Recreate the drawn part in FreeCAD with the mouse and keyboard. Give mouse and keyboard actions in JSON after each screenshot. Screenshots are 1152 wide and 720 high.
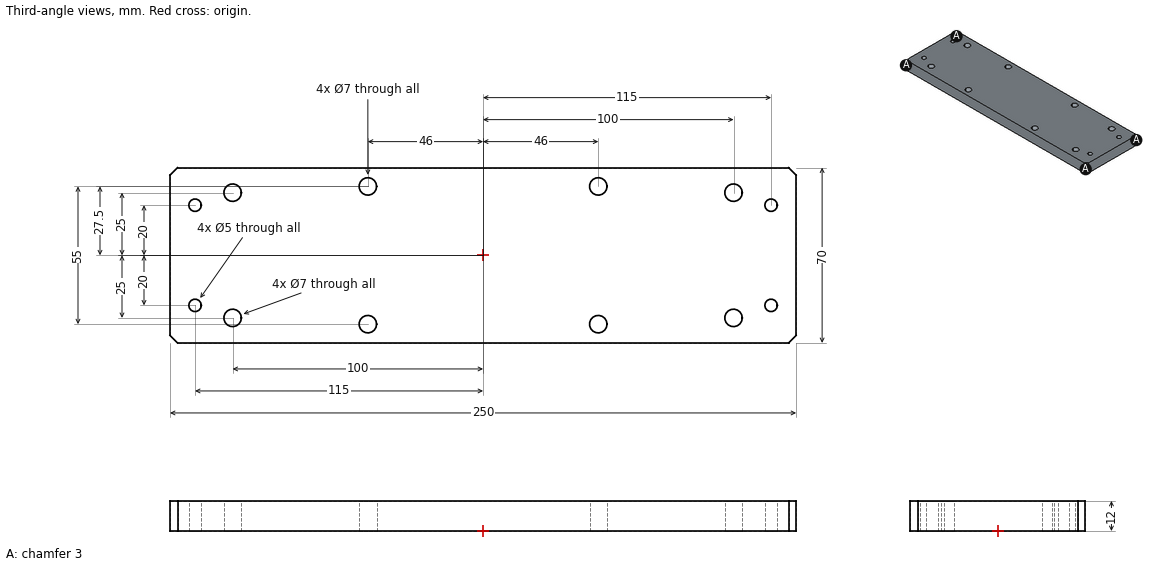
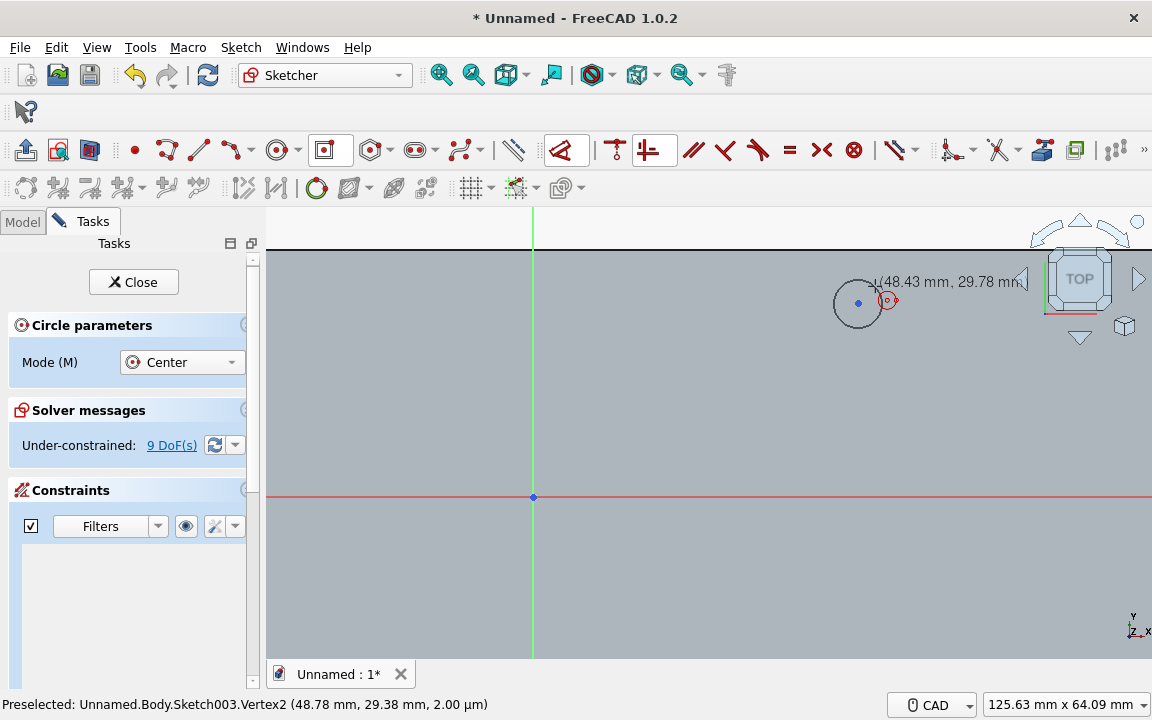
{"action": "scroll", "coordinate": [858, 303], "scroll_direction": "down", "scroll_amount": 2}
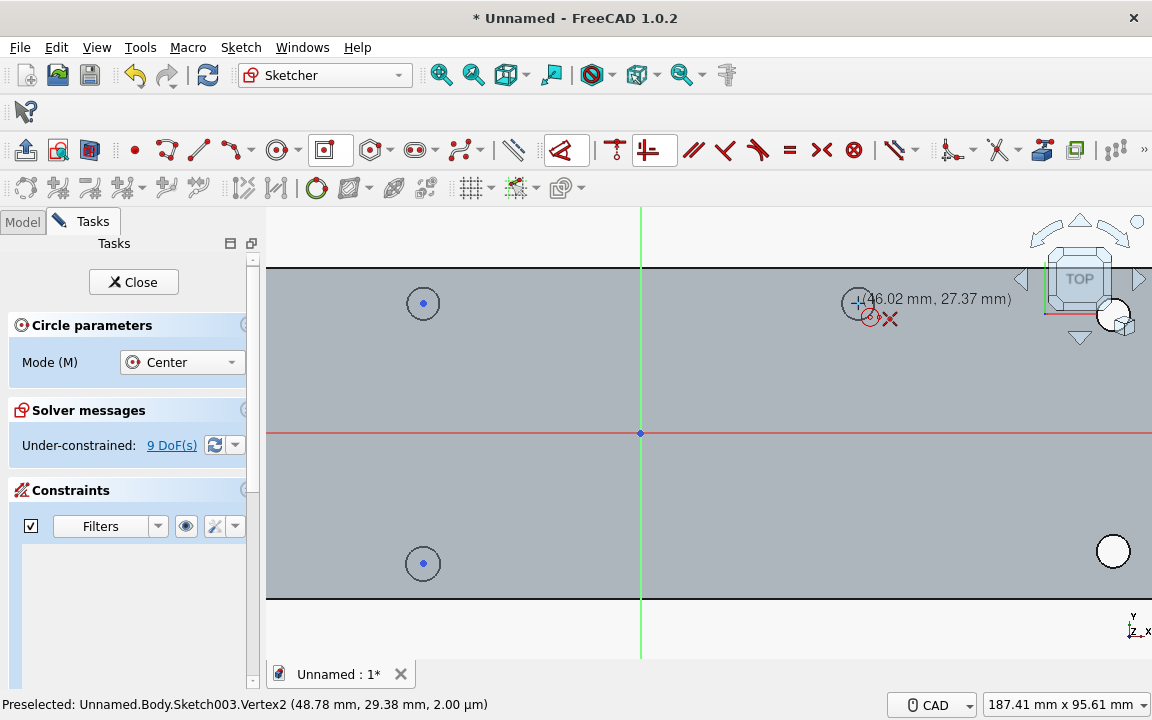
{"action": "scroll", "coordinate": [858, 563], "scroll_direction": "up", "scroll_amount": 2}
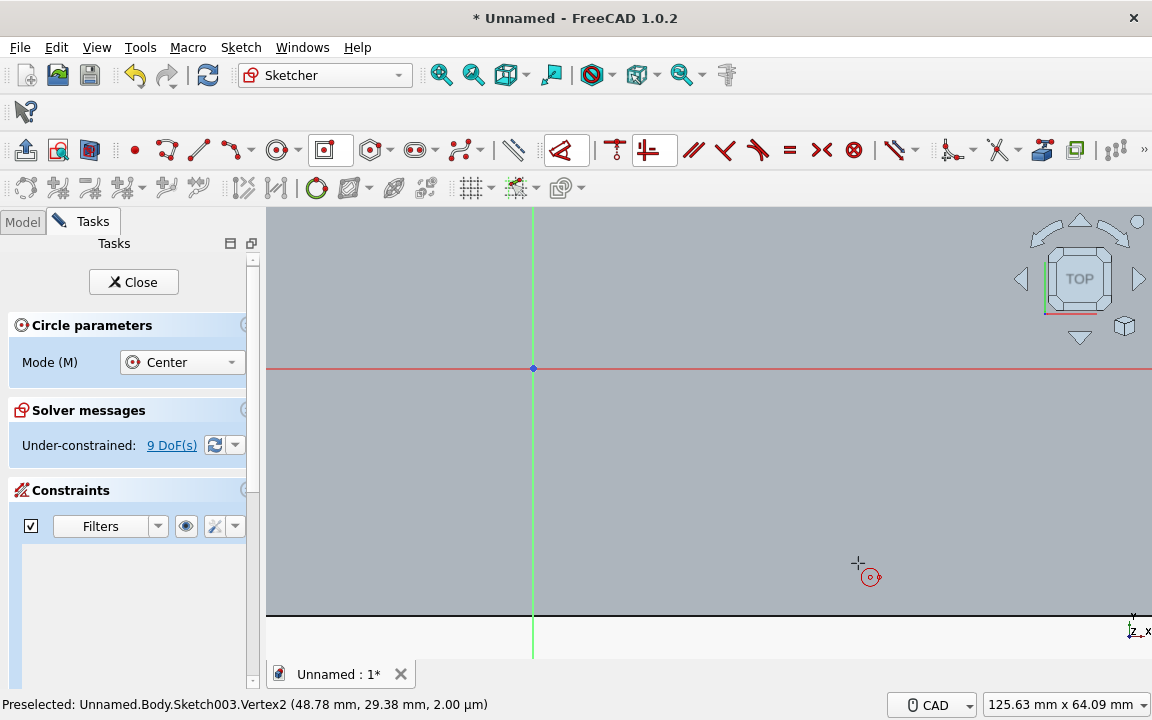
{"action": "left_click", "coordinate": [858, 563]}
{"action": "left_click", "coordinate": [875, 545]}
{"action": "key", "text": "Escape"}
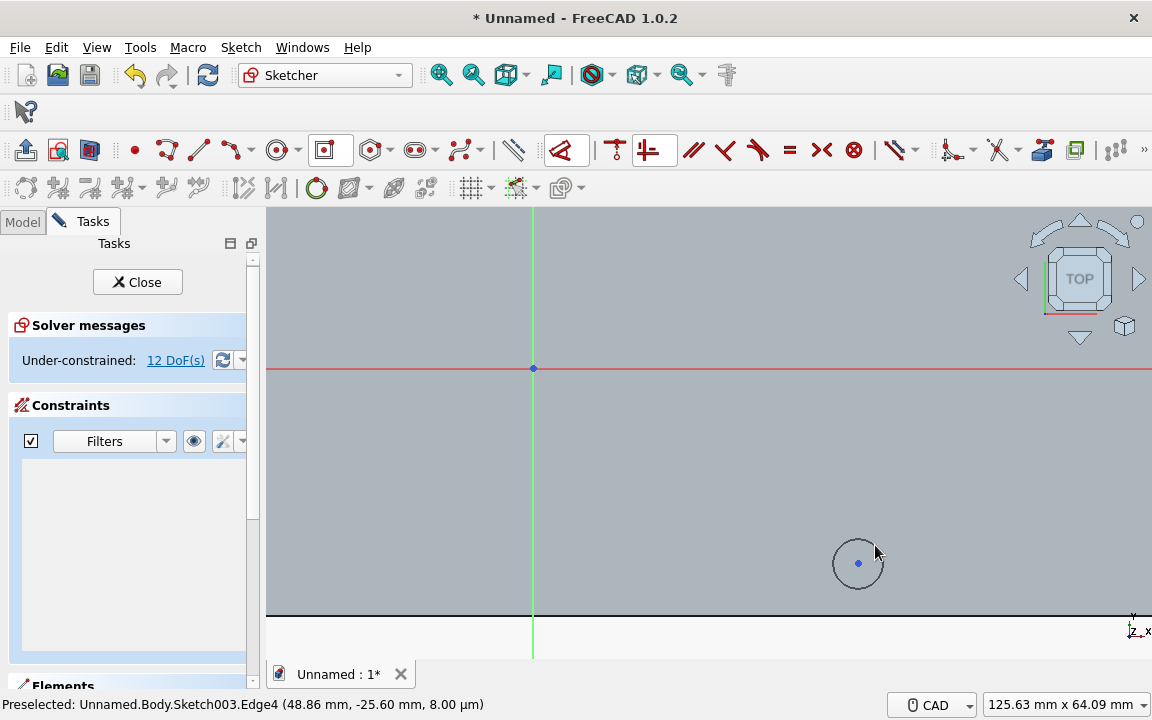
{"action": "scroll", "coordinate": [858, 563], "scroll_direction": "down", "scroll_amount": 2}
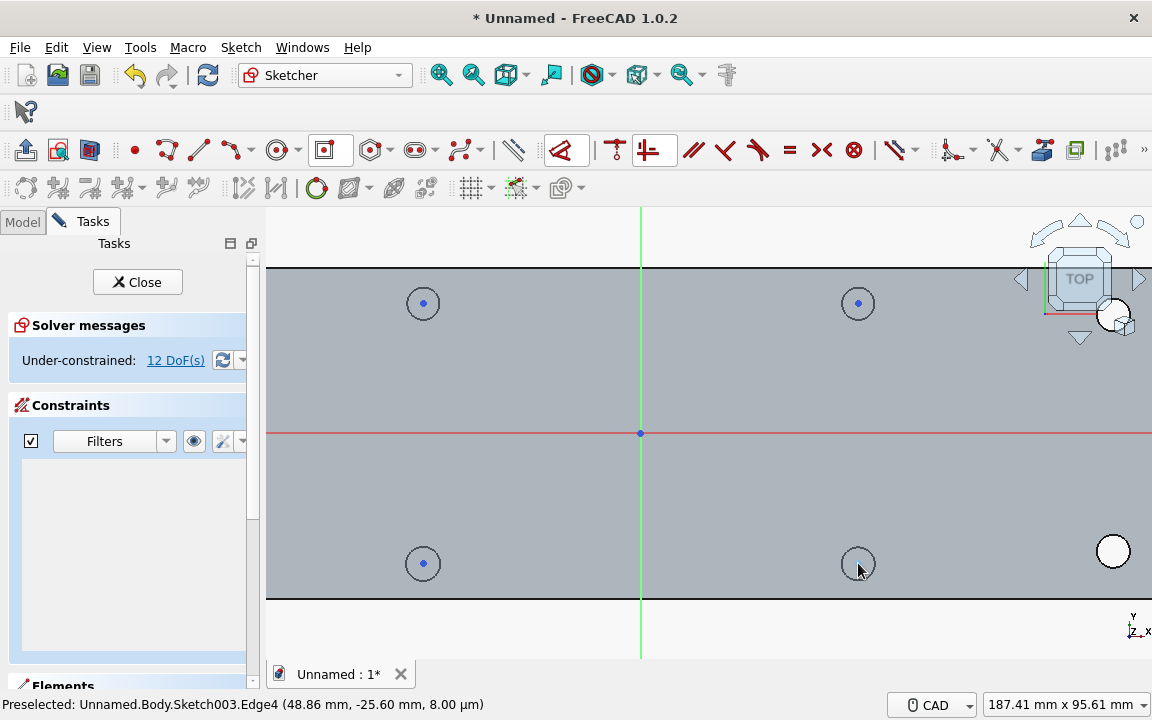
{"action": "left_click", "coordinate": [435, 292]}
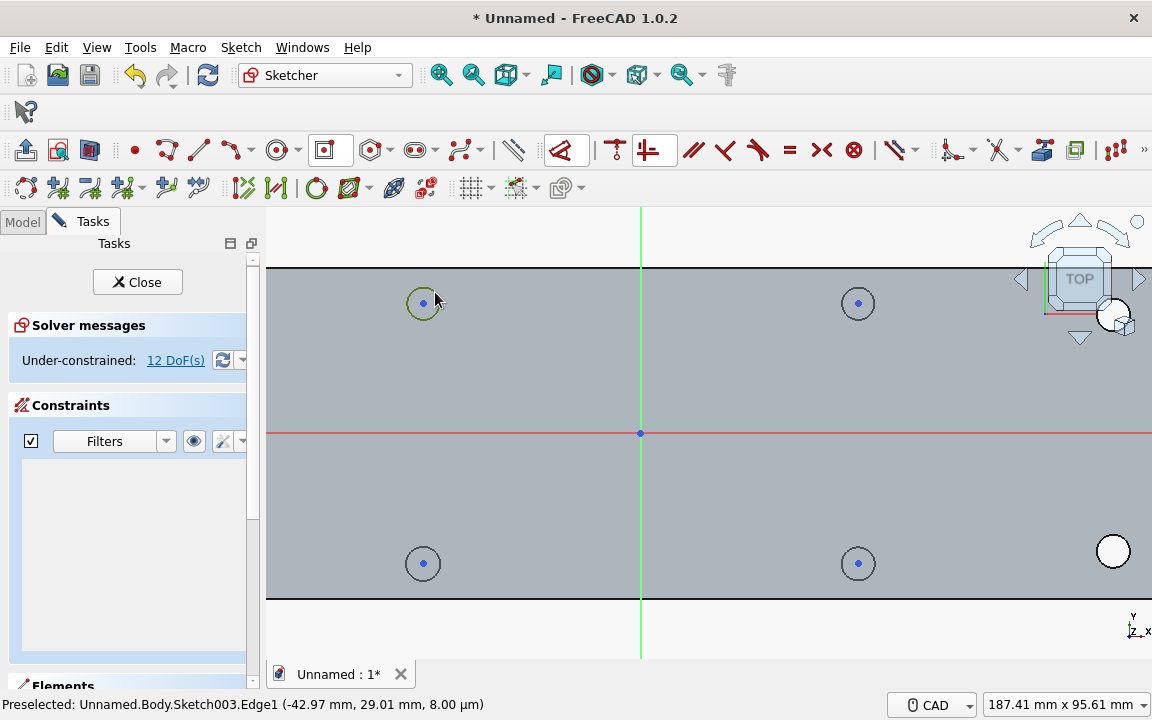
{"action": "left_click", "coordinate": [435, 552]}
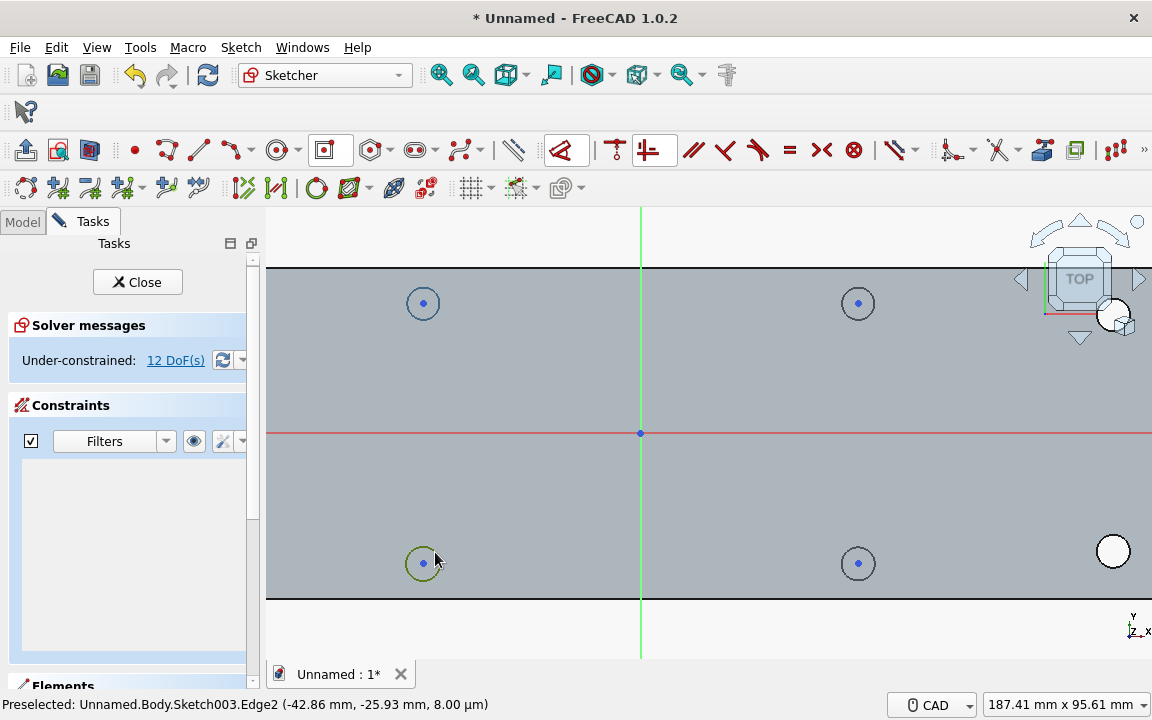
{"action": "left_click", "coordinate": [870, 292]}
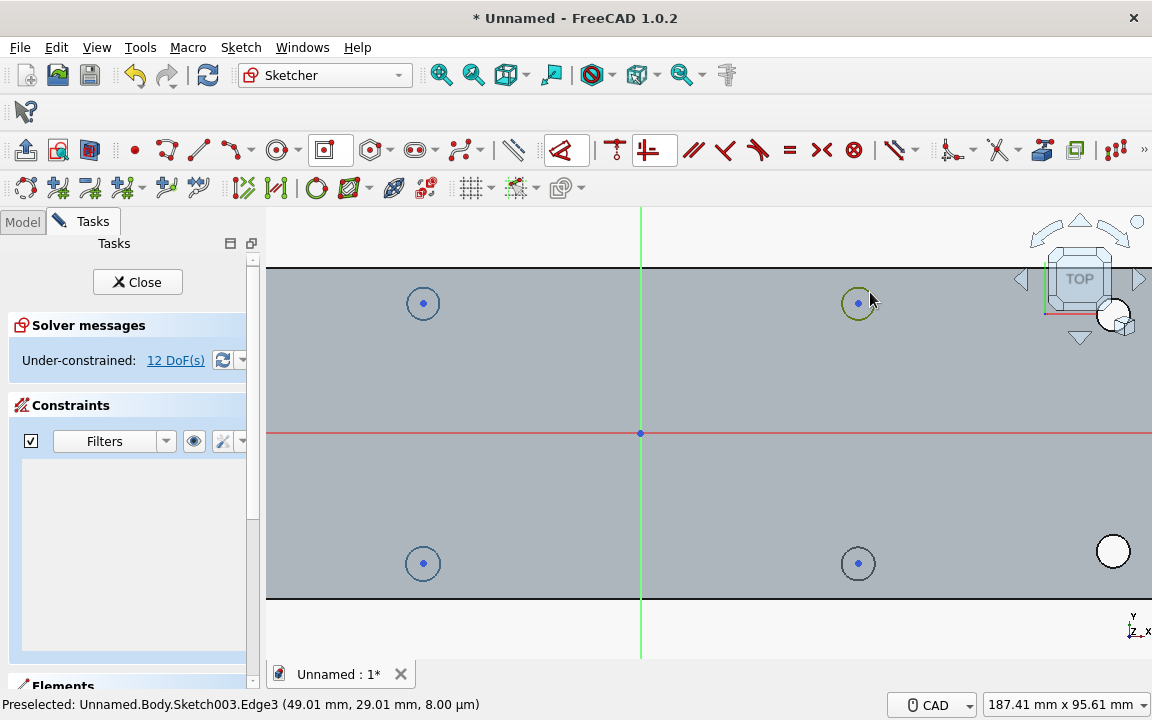
{"action": "left_click", "coordinate": [870, 552]}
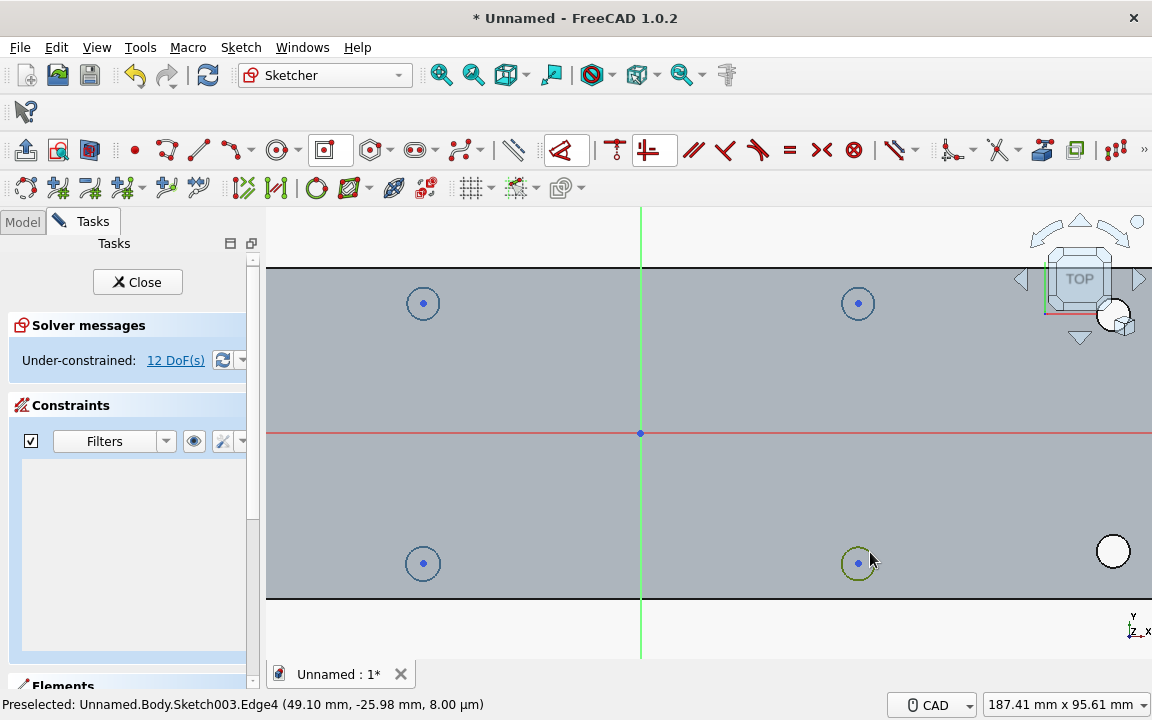
{"action": "left_click", "coordinate": [790, 150]}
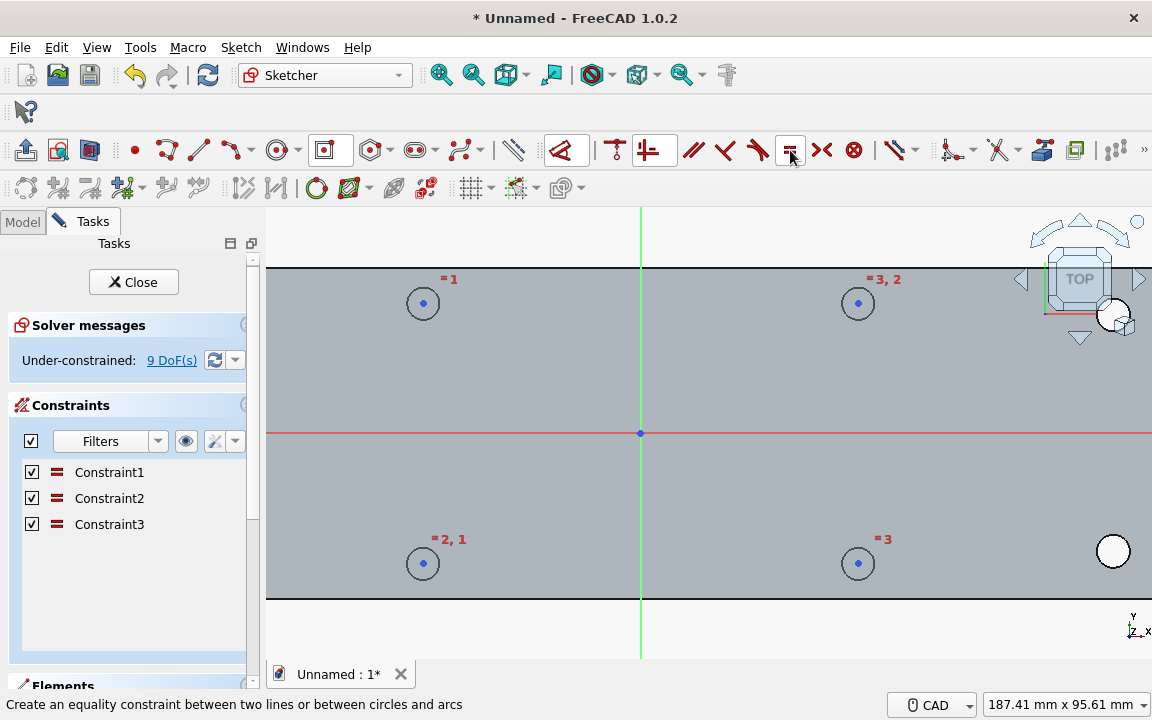
{"action": "left_click", "coordinate": [423, 304]}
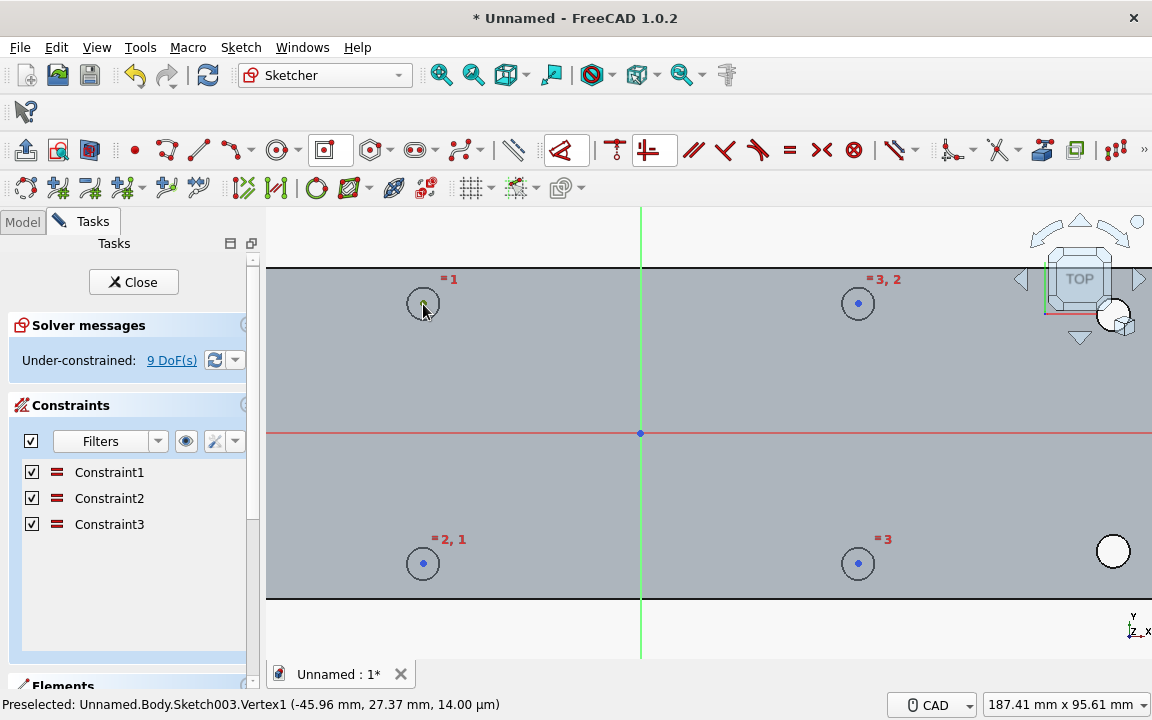
{"action": "left_click", "coordinate": [423, 564]}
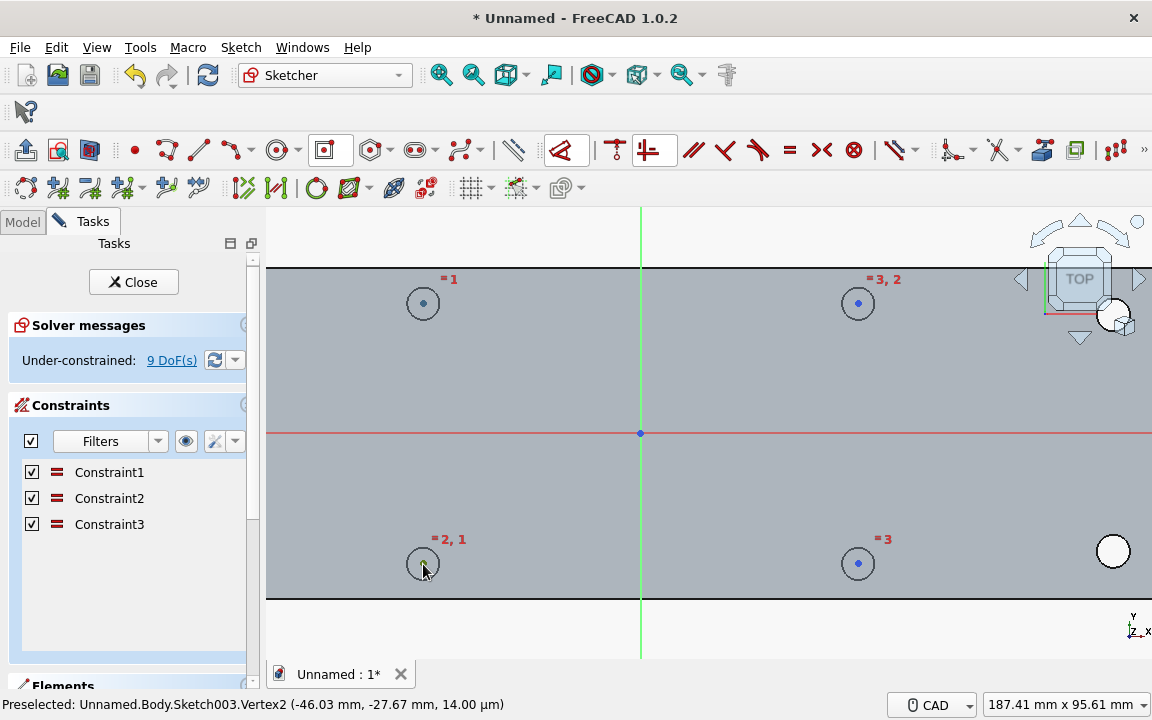
{"action": "key", "text": "v"}